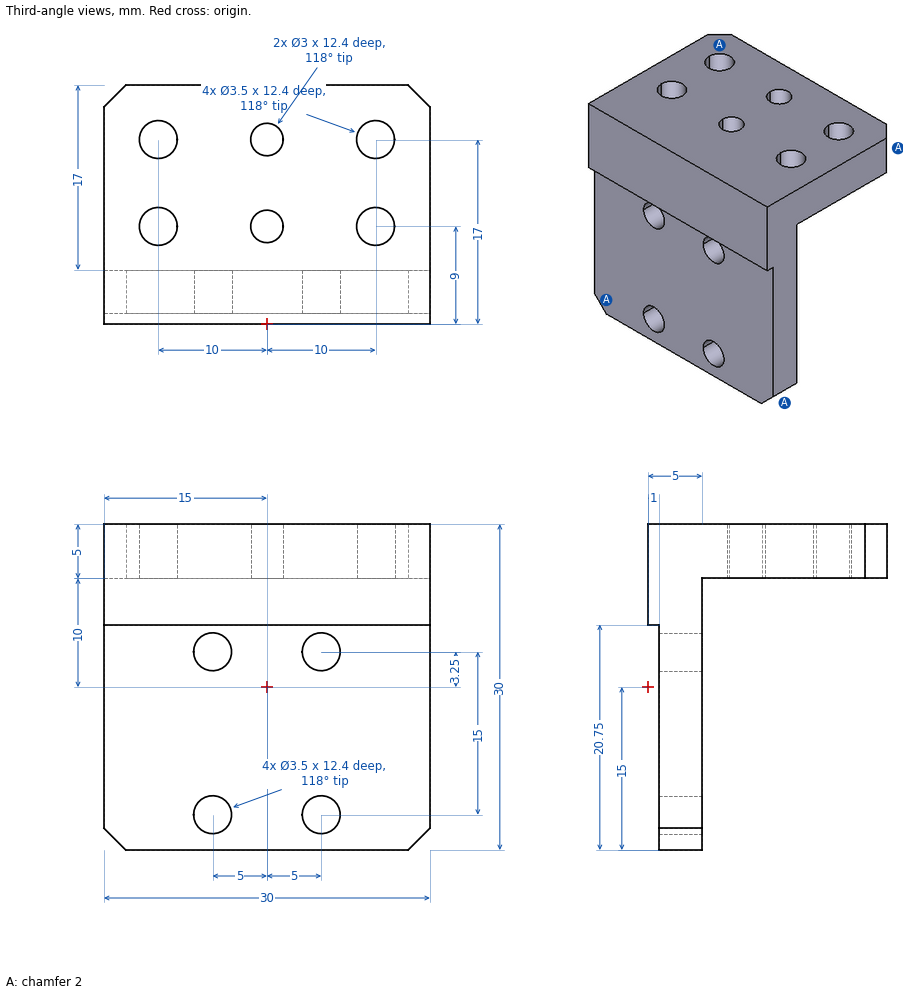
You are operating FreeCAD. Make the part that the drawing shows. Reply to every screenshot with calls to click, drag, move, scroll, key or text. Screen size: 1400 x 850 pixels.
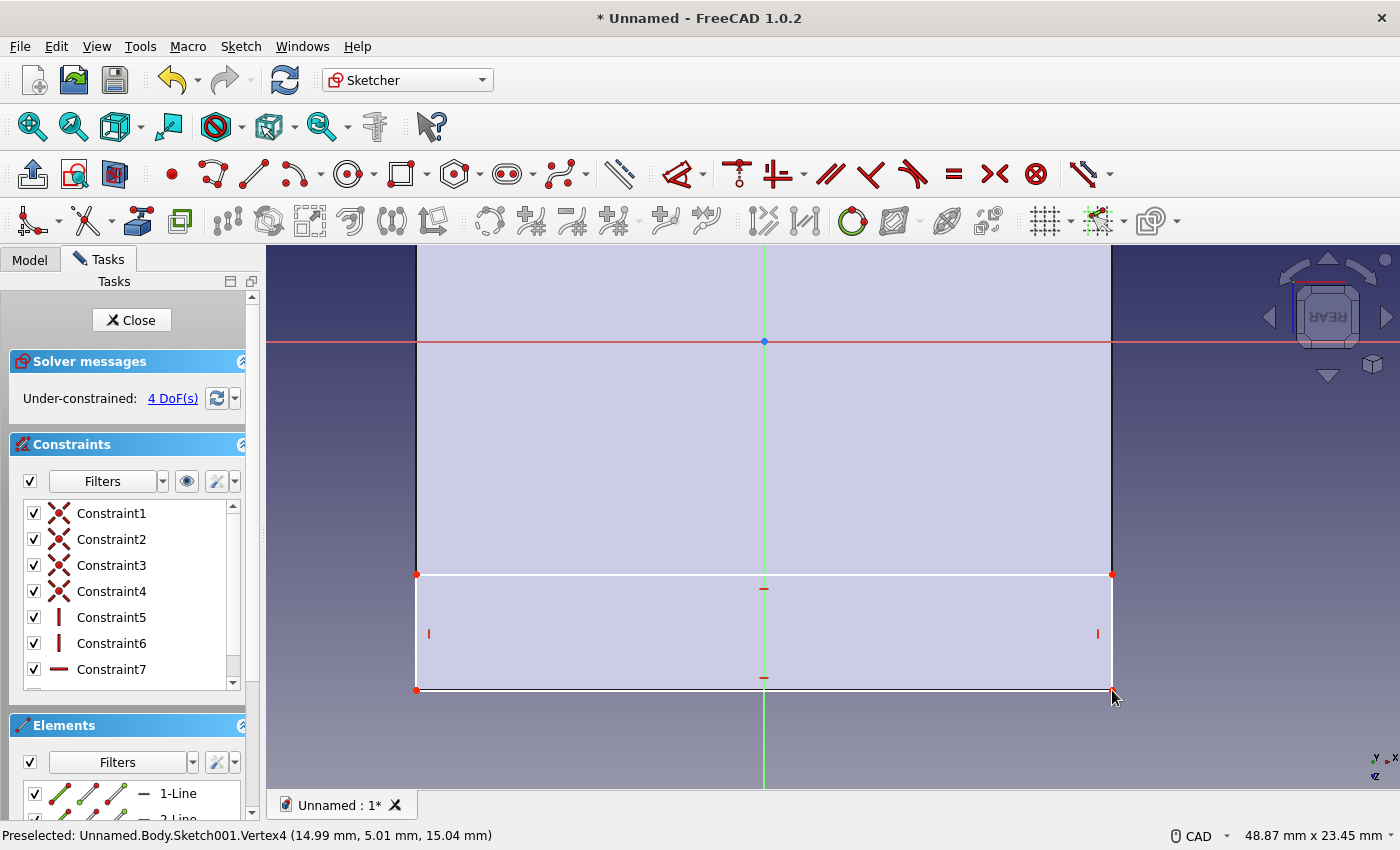
key(d)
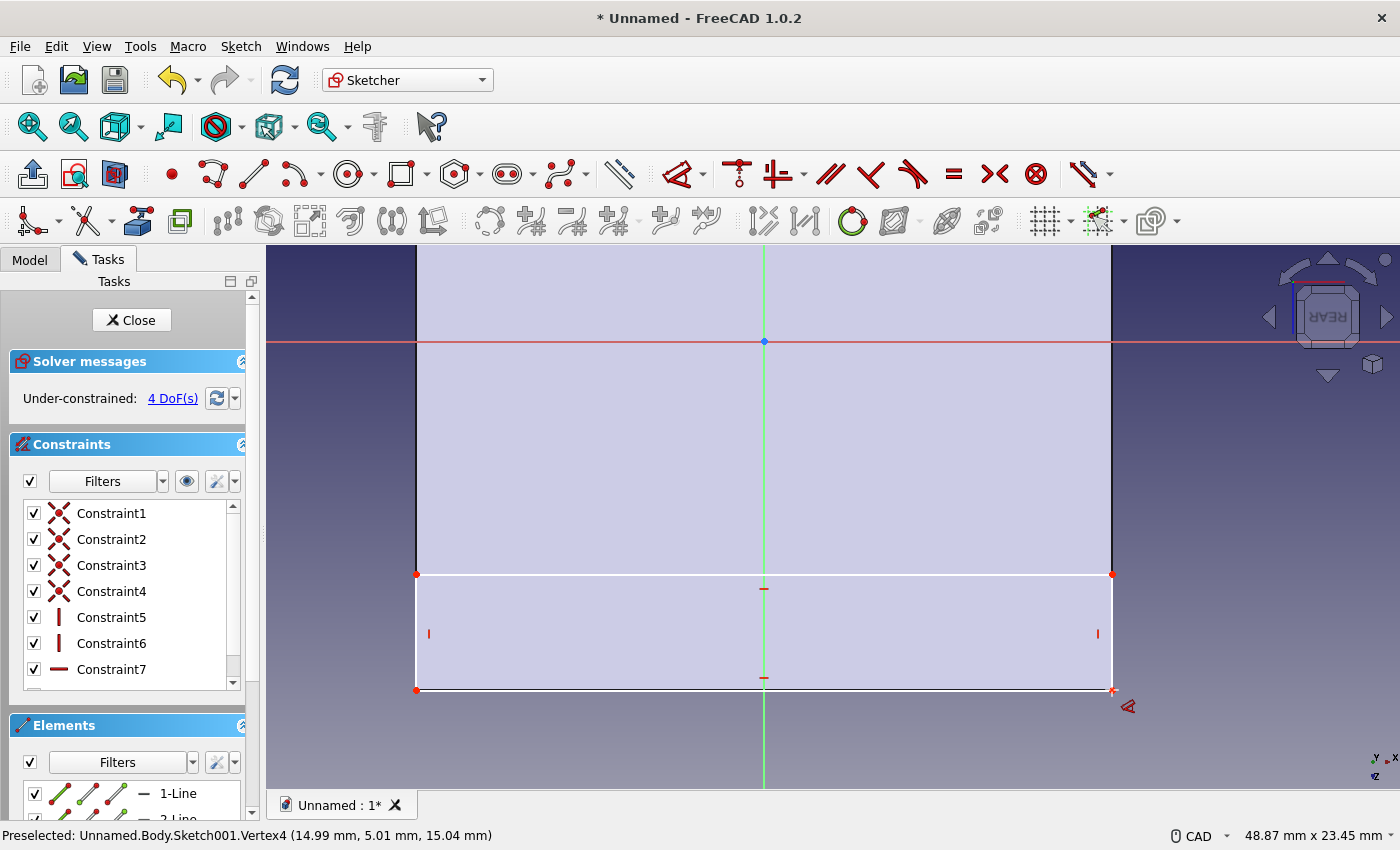
click(416, 610)
click(382, 633)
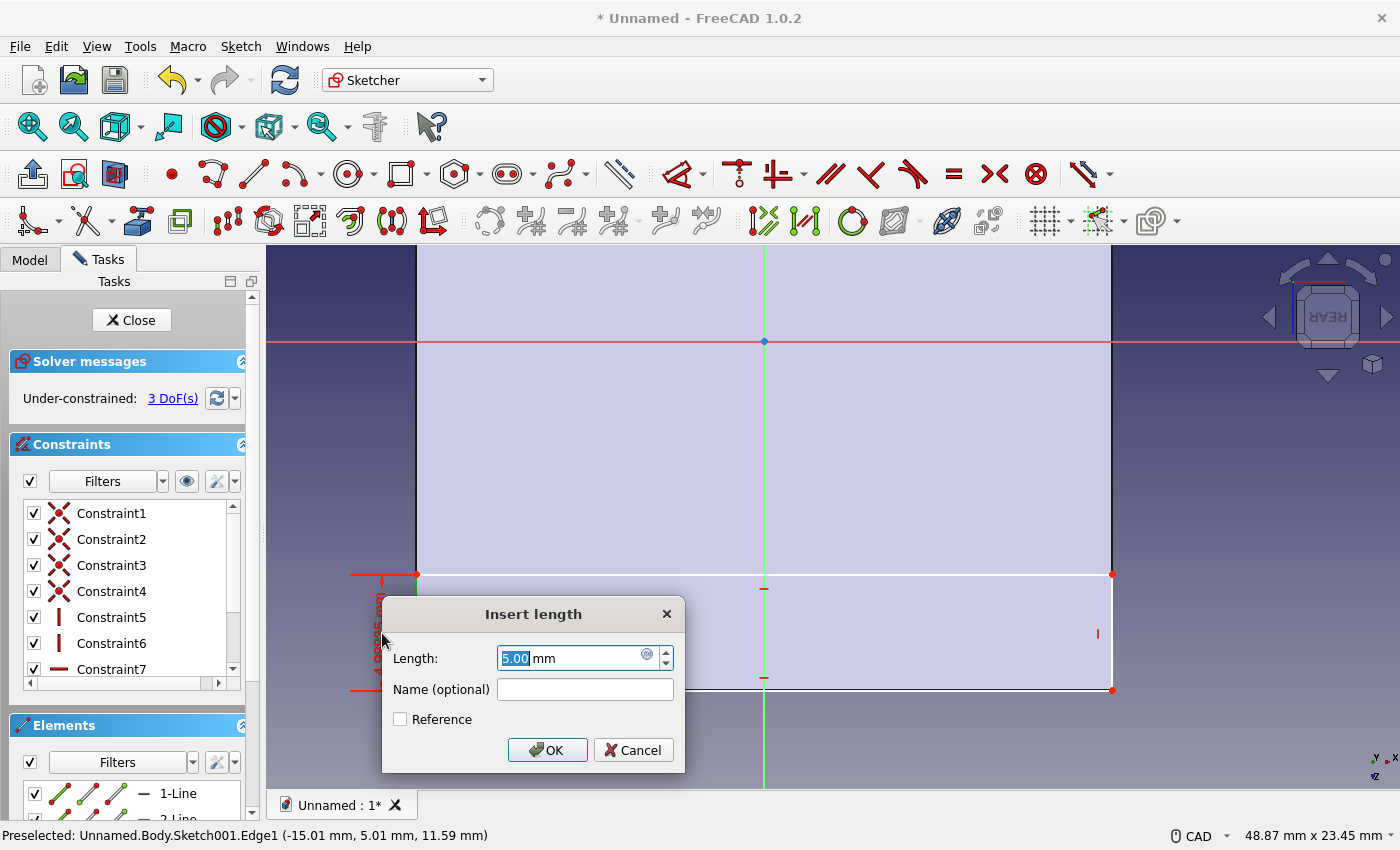
text(5)
key(Return)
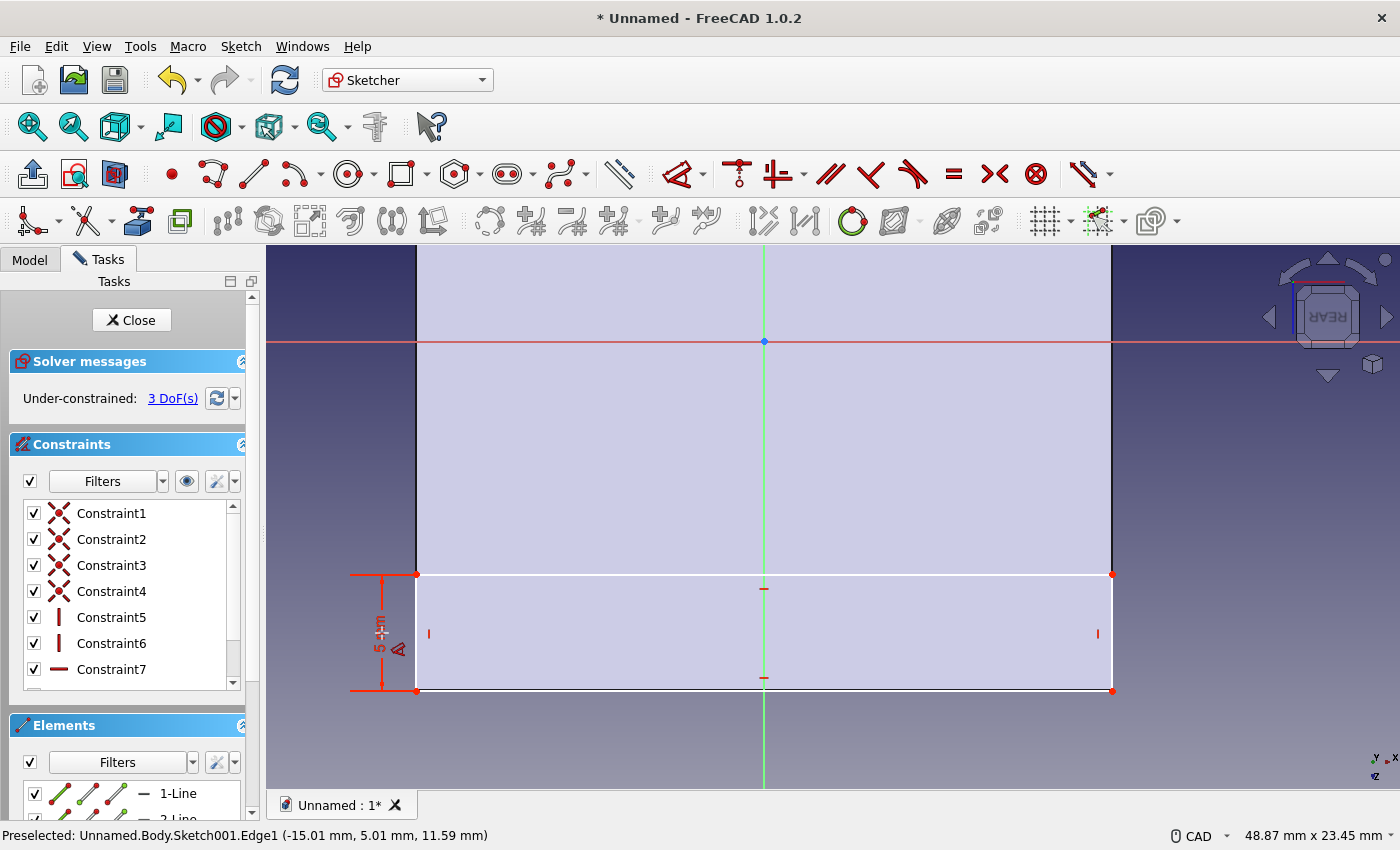
click(625, 691)
click(604, 725)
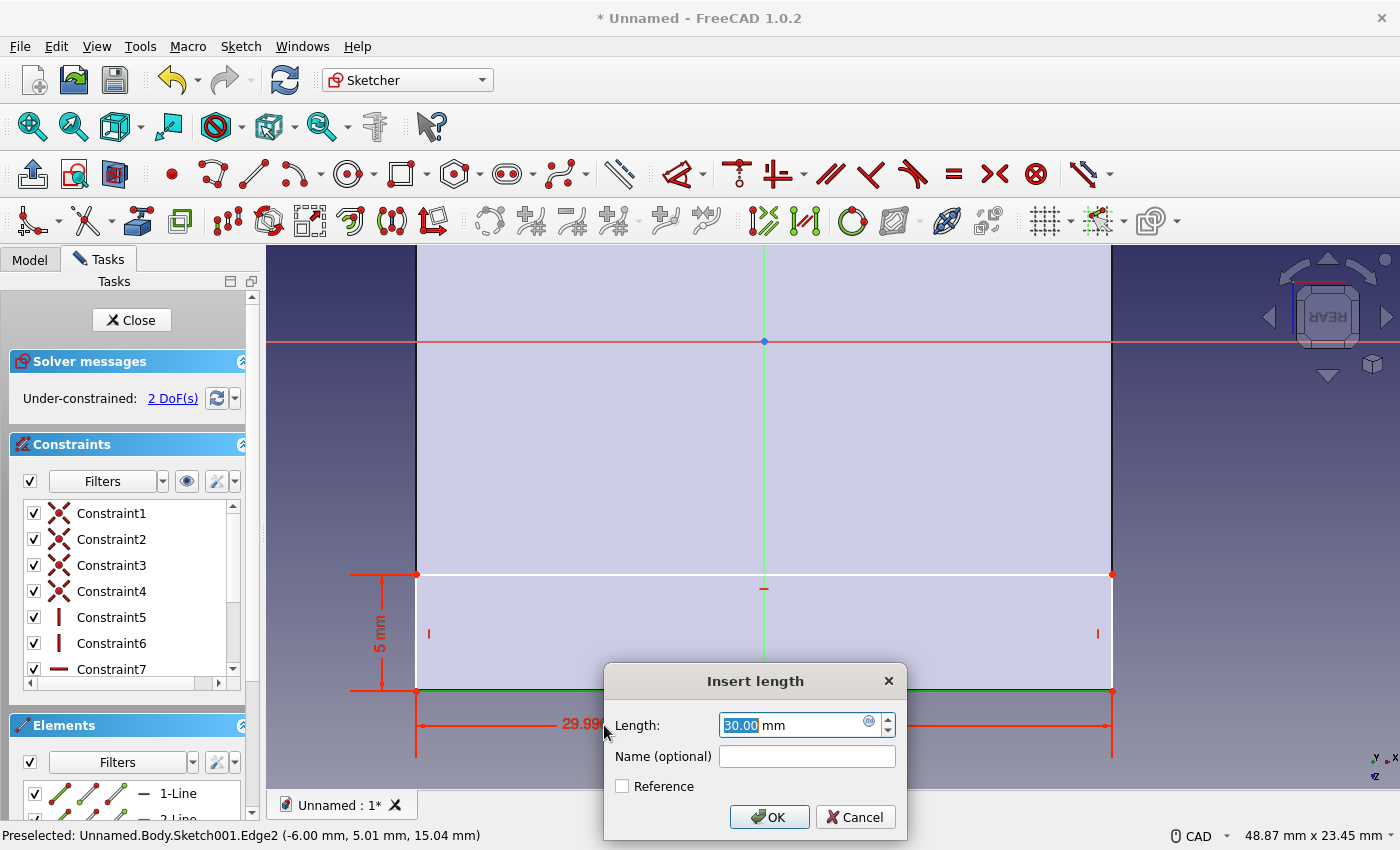
text(30)
key(Return)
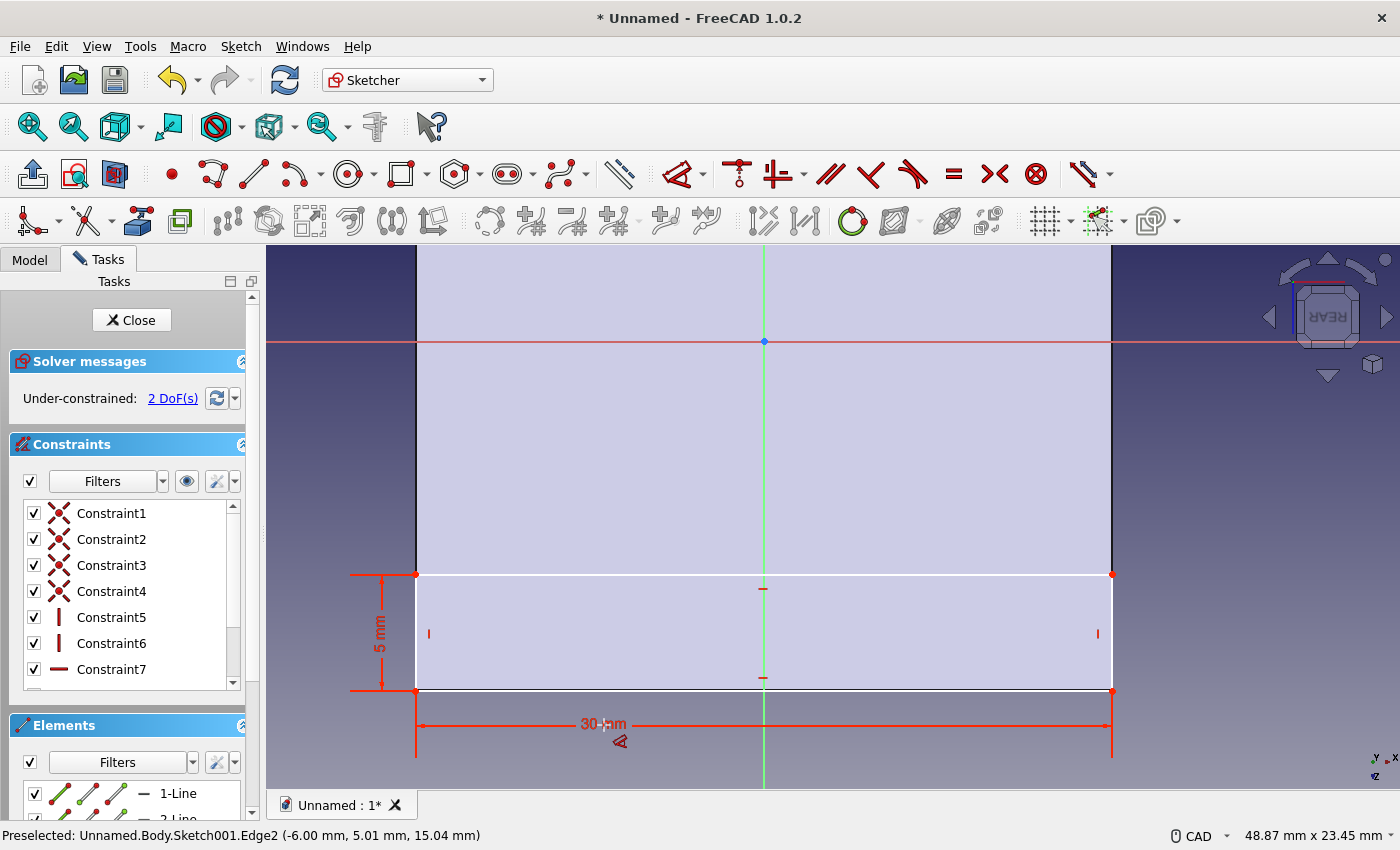
click(416, 575)
click(590, 308)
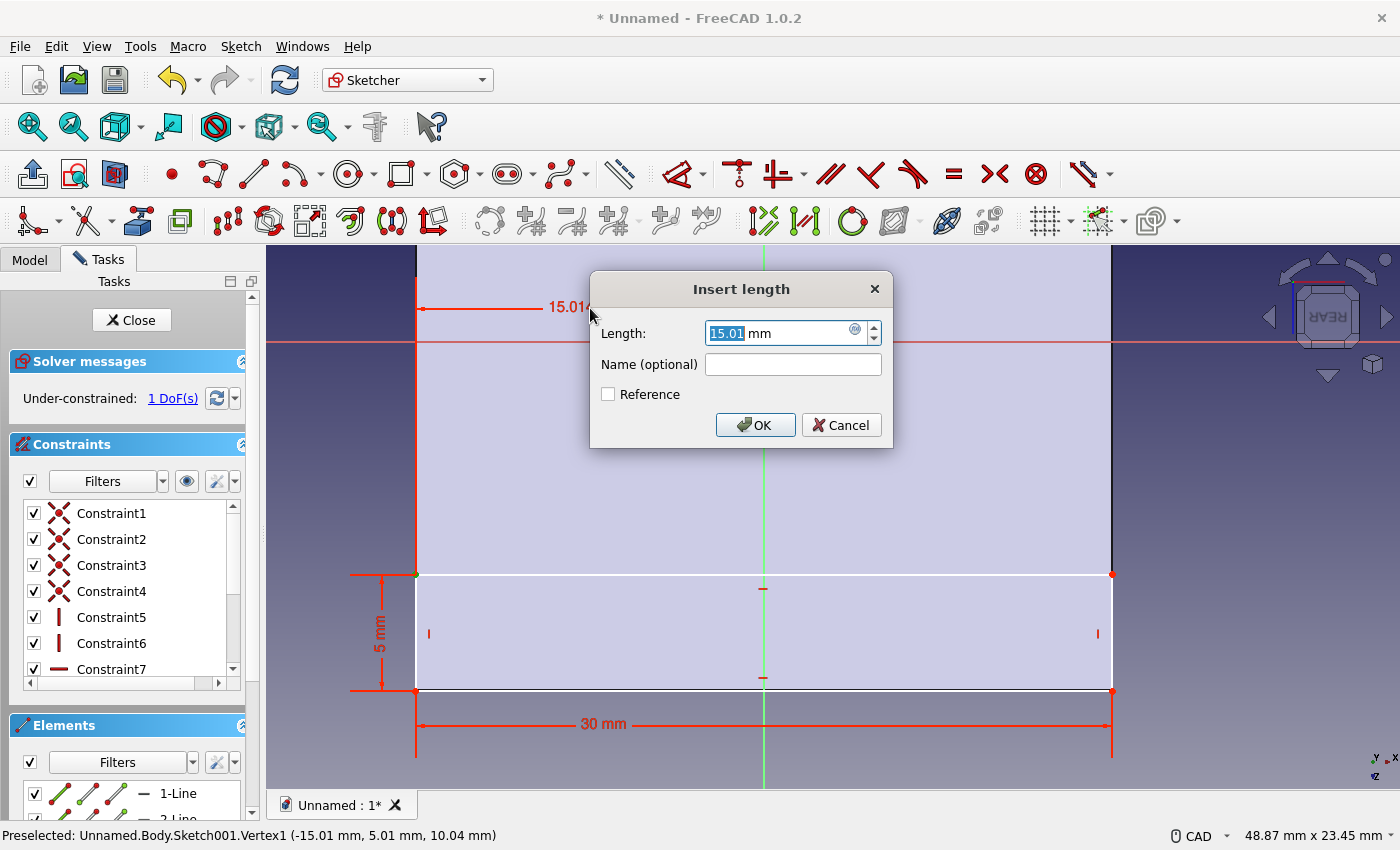
text(15)
key(Return)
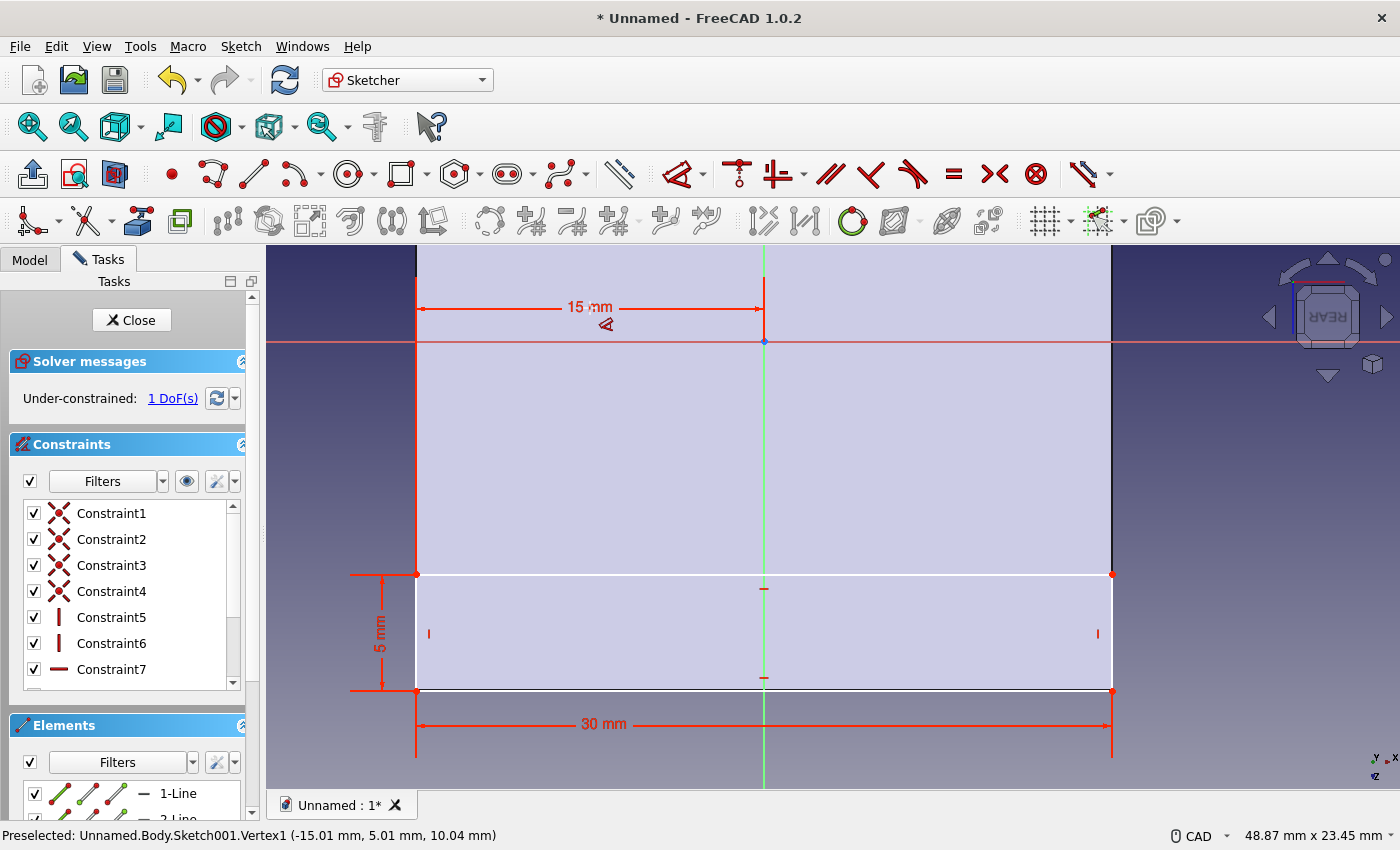
click(416, 575)
click(382, 458)